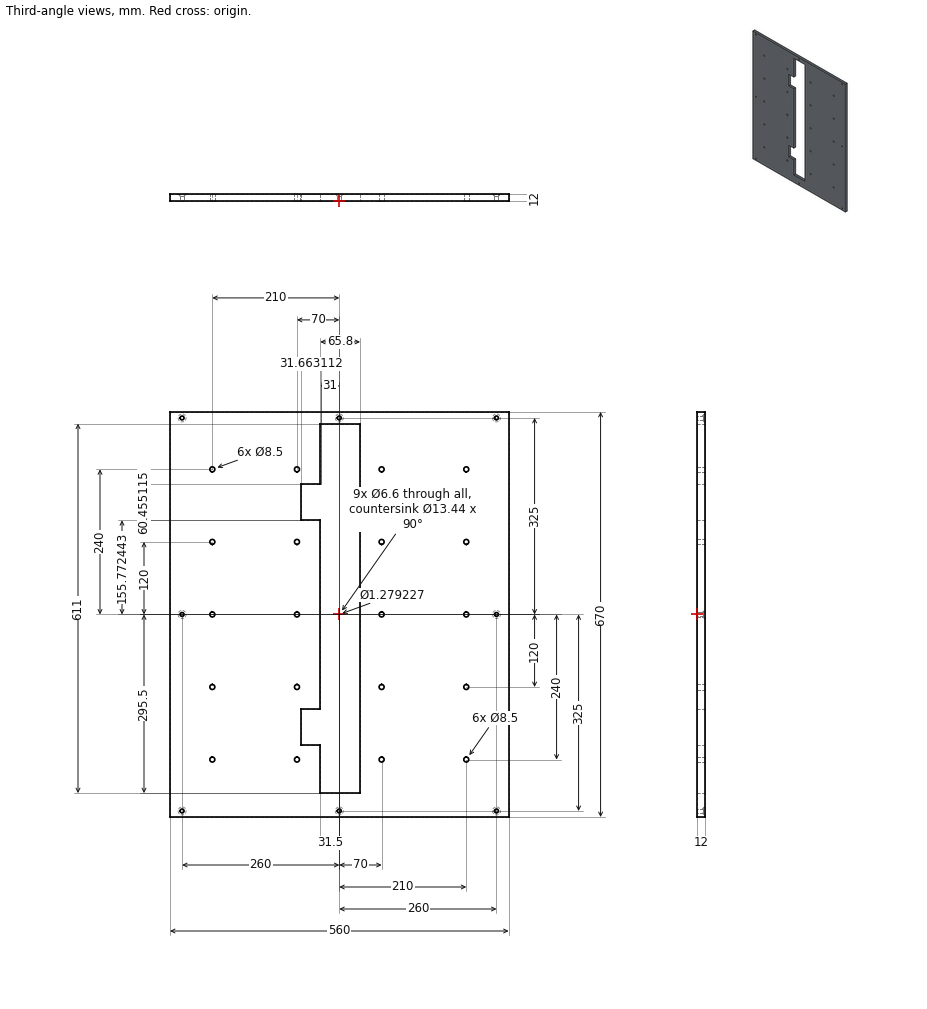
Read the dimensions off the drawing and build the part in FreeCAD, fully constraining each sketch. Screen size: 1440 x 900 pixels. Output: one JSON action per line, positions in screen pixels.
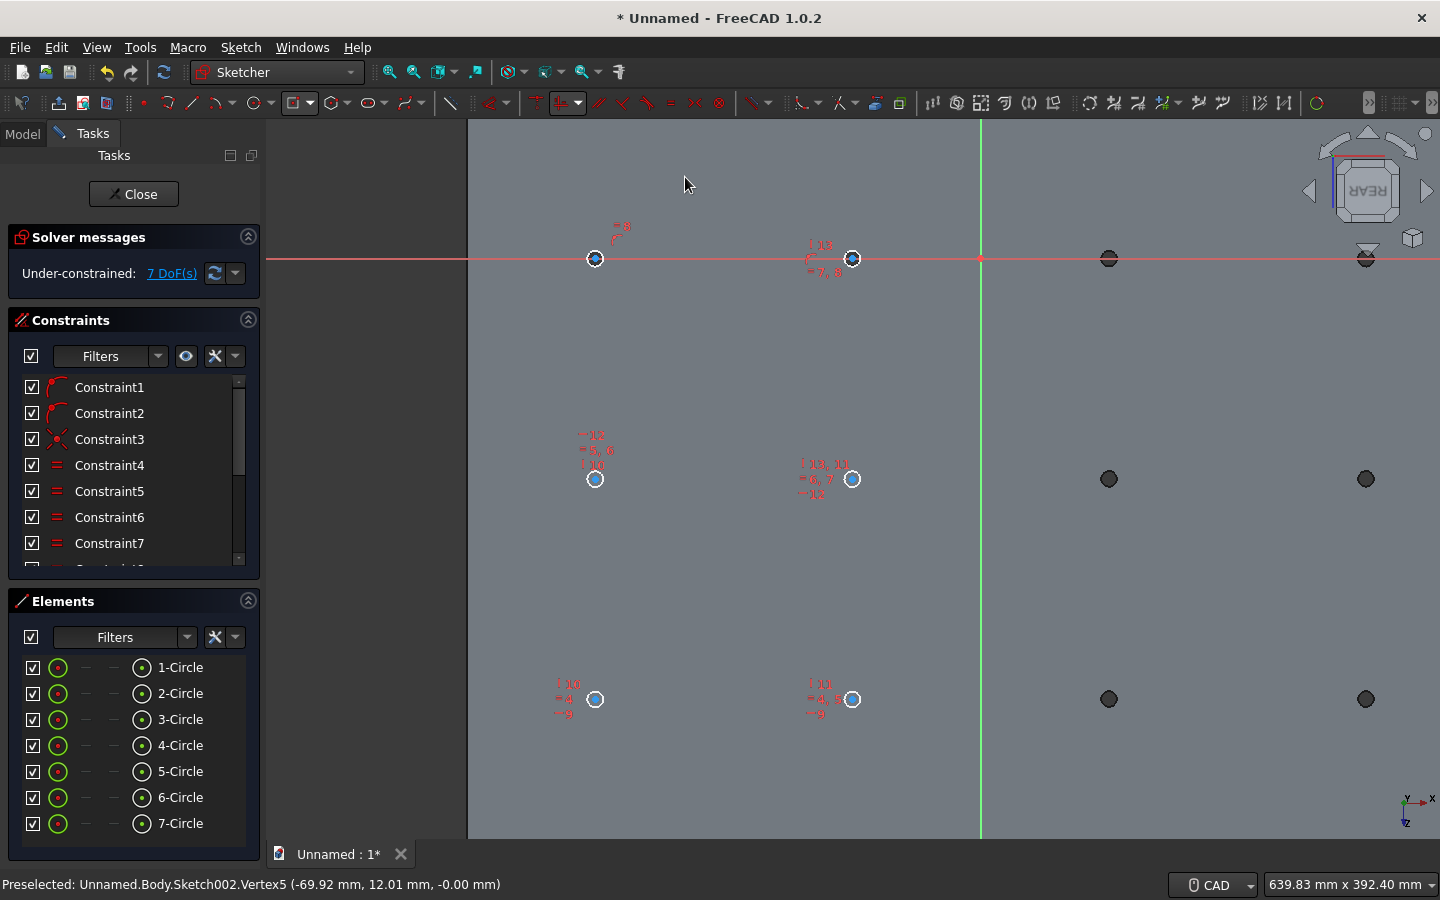
{"action": "left_click", "coordinate": [595, 479]}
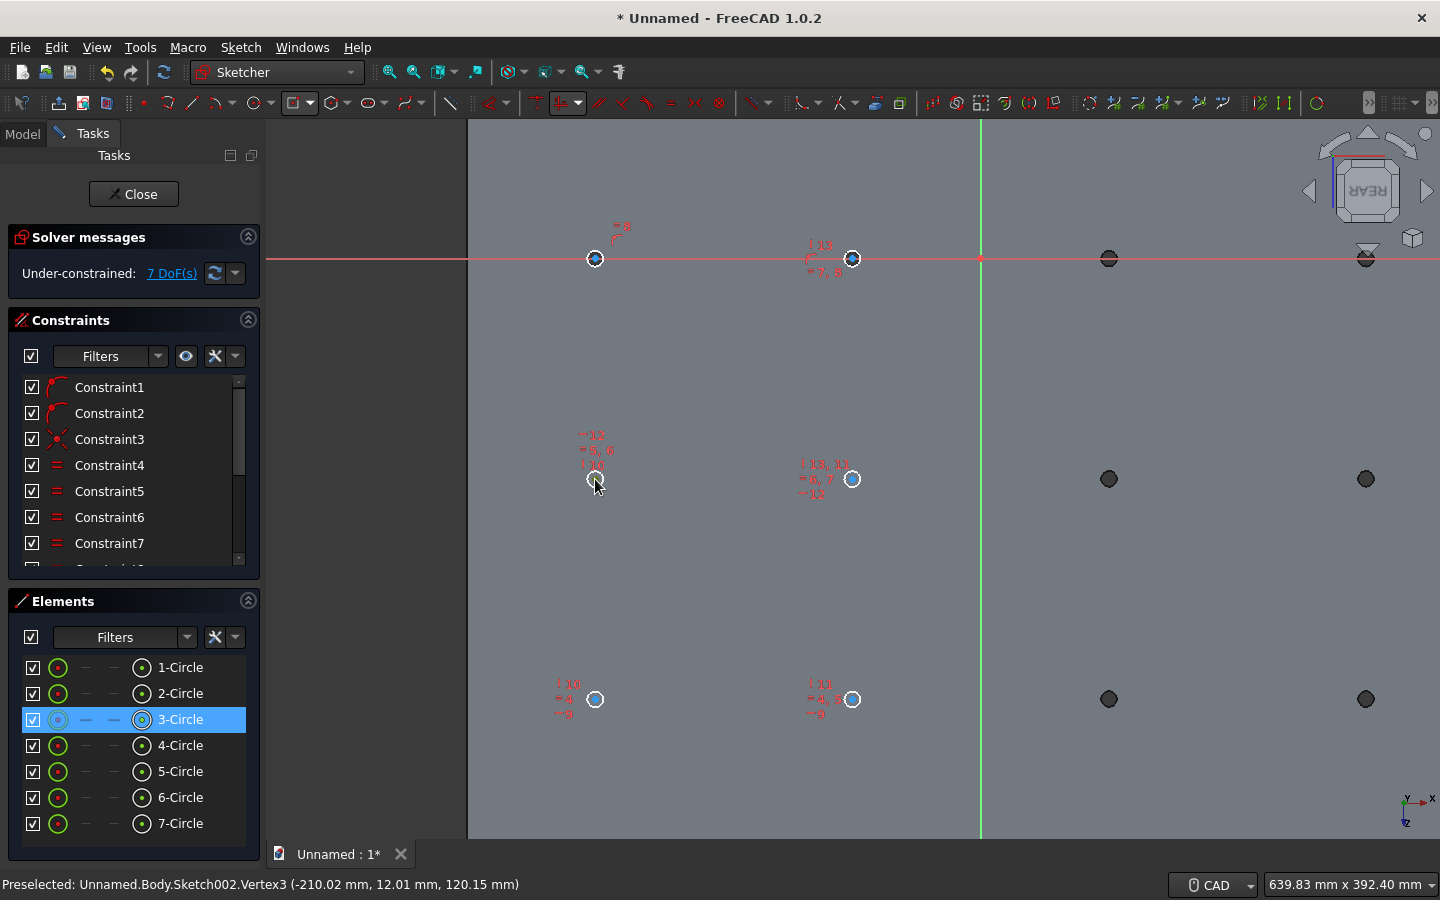
{"action": "left_click", "coordinate": [595, 259]}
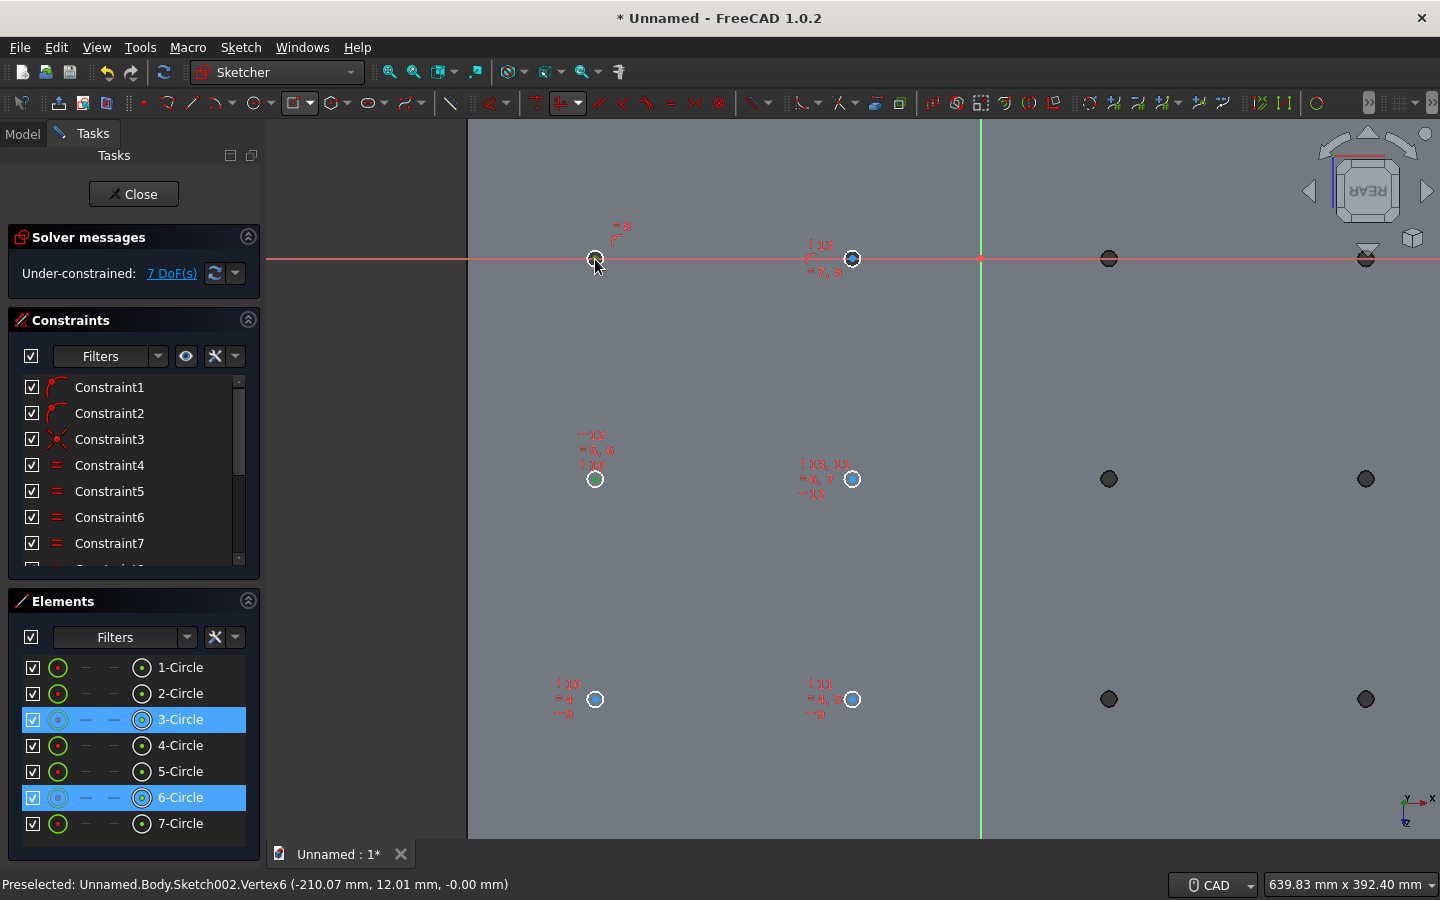
{"action": "left_click", "coordinate": [580, 104]}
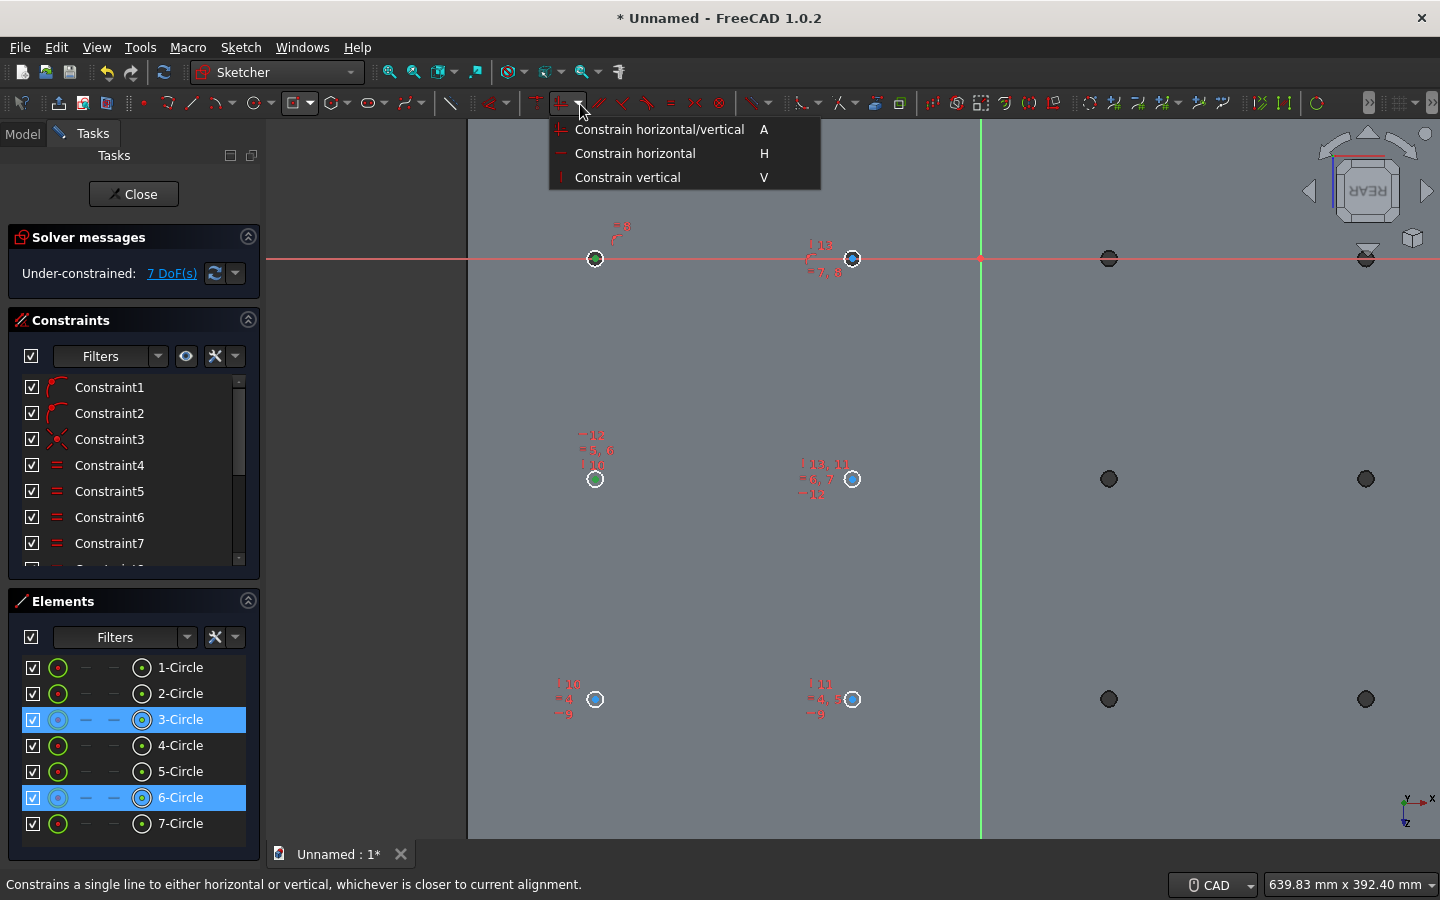
{"action": "left_click", "coordinate": [685, 177]}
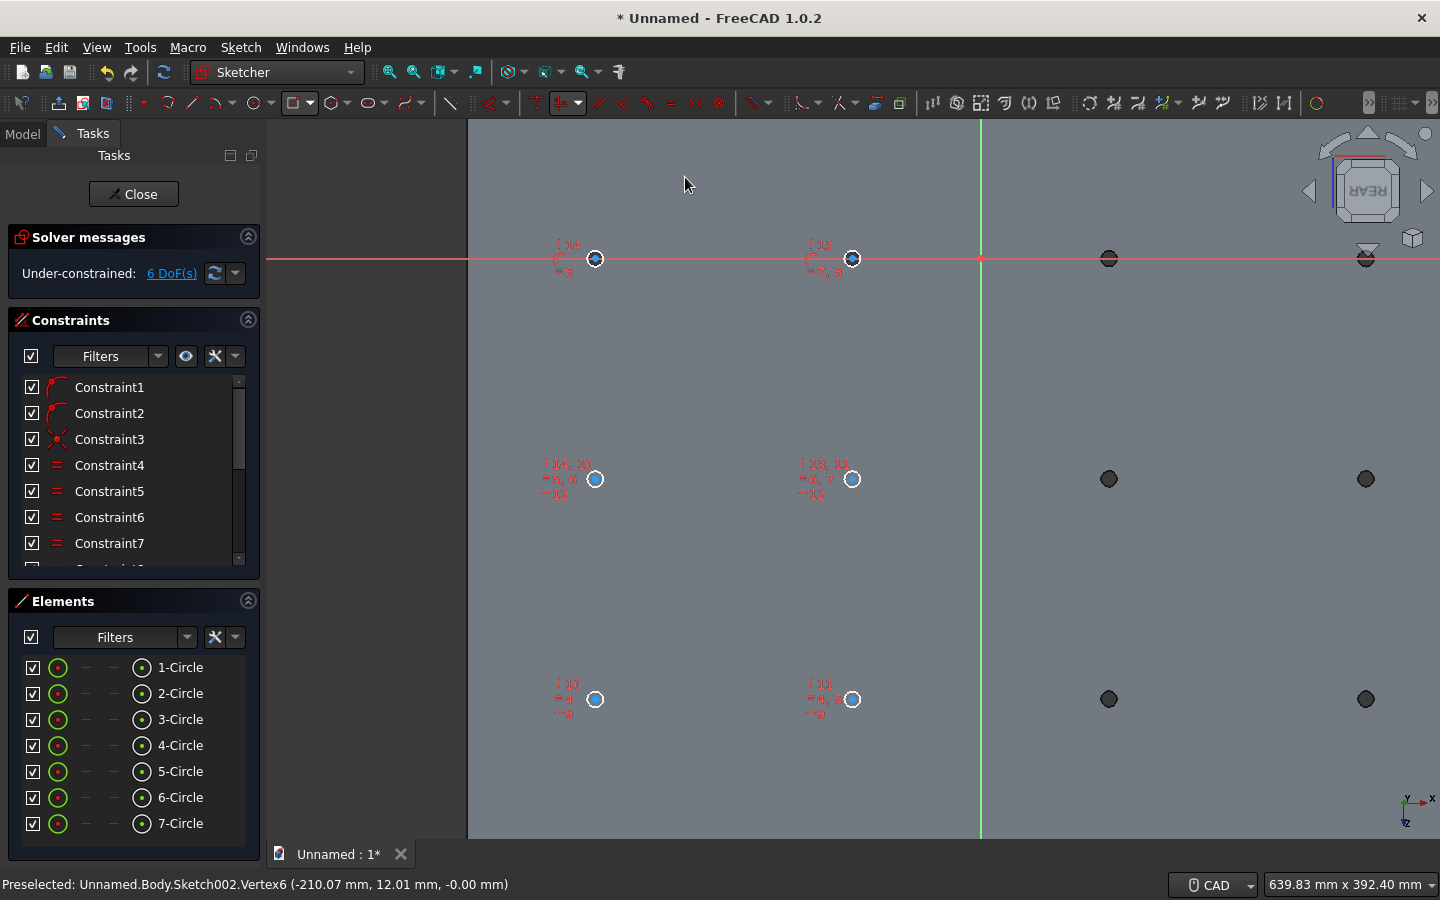
{"action": "left_click", "coordinate": [490, 104]}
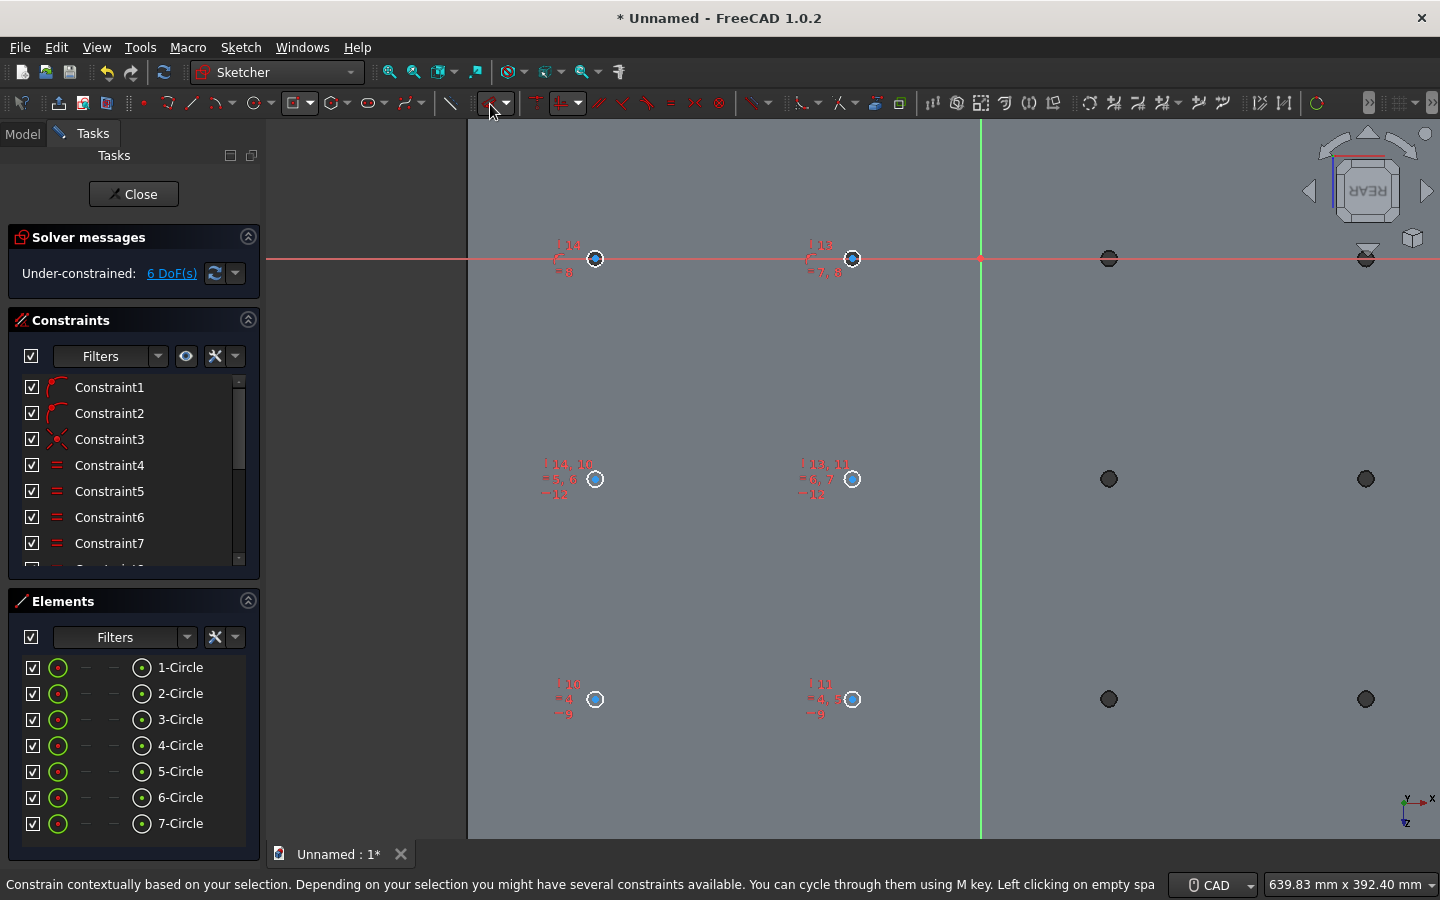
{"action": "scroll", "coordinate": [601, 694], "scroll_direction": "up", "scroll_amount": 5}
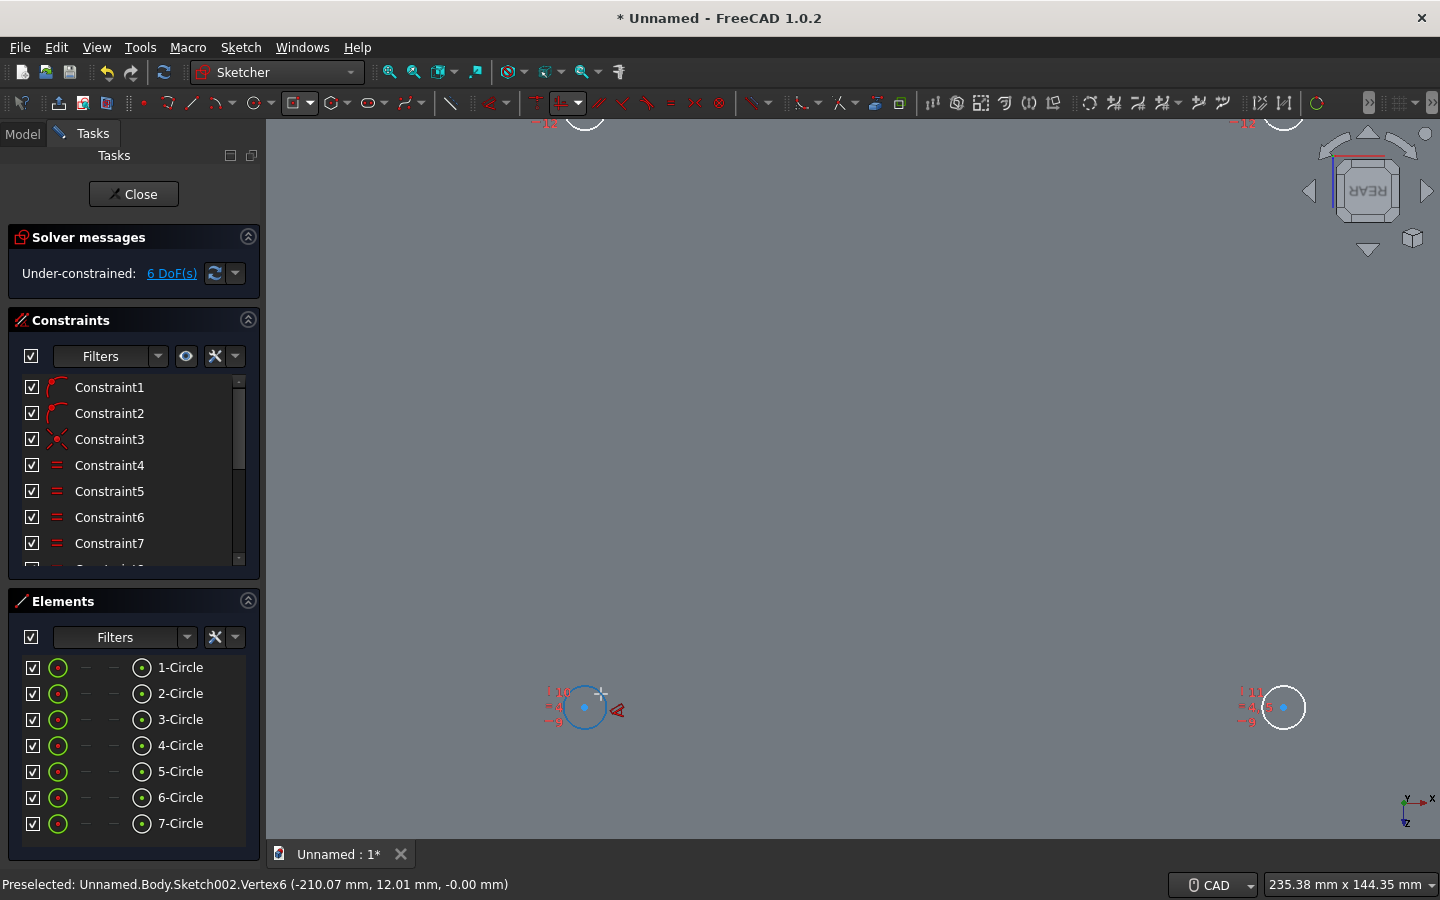
{"action": "left_click", "coordinate": [600, 692]}
{"action": "left_click", "coordinate": [622, 669]}